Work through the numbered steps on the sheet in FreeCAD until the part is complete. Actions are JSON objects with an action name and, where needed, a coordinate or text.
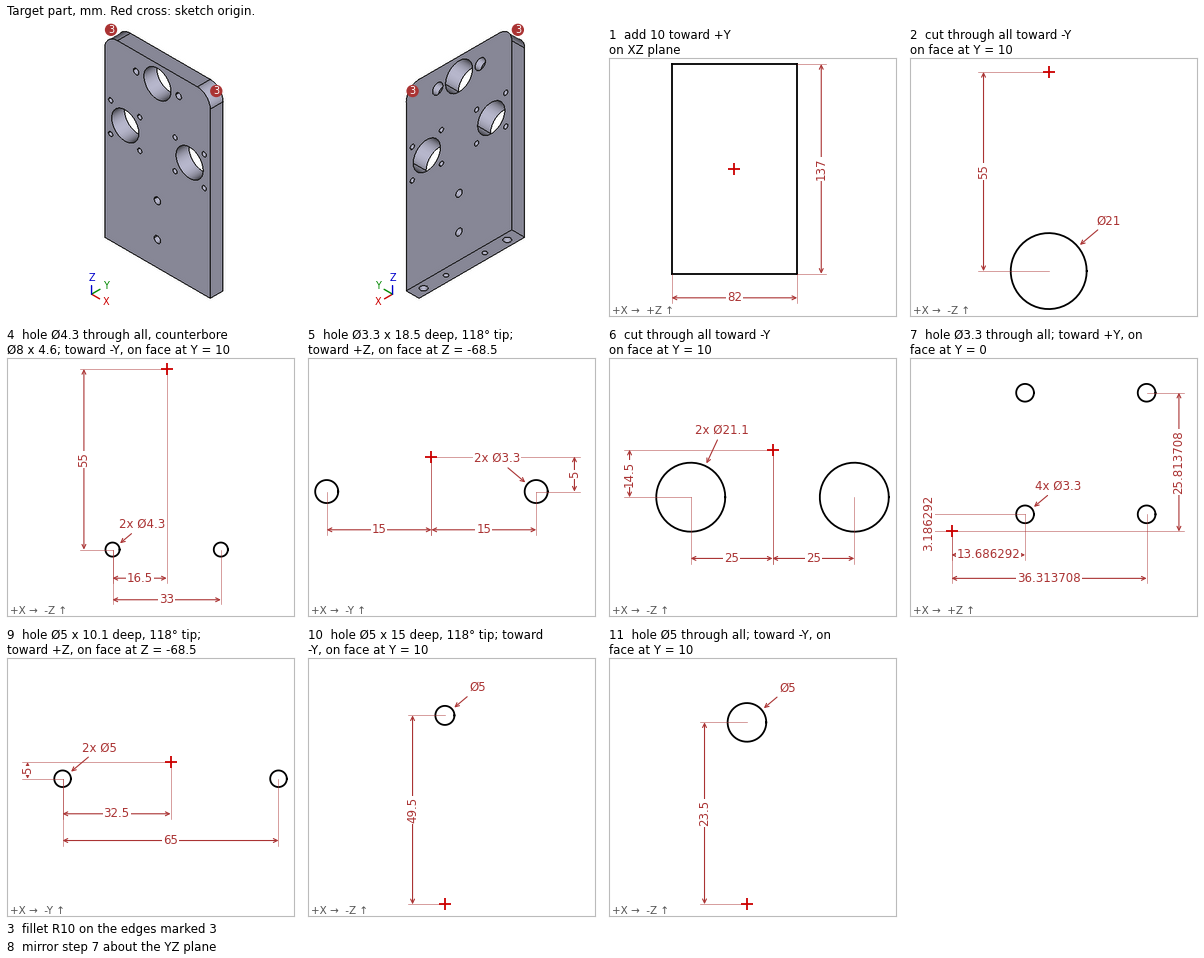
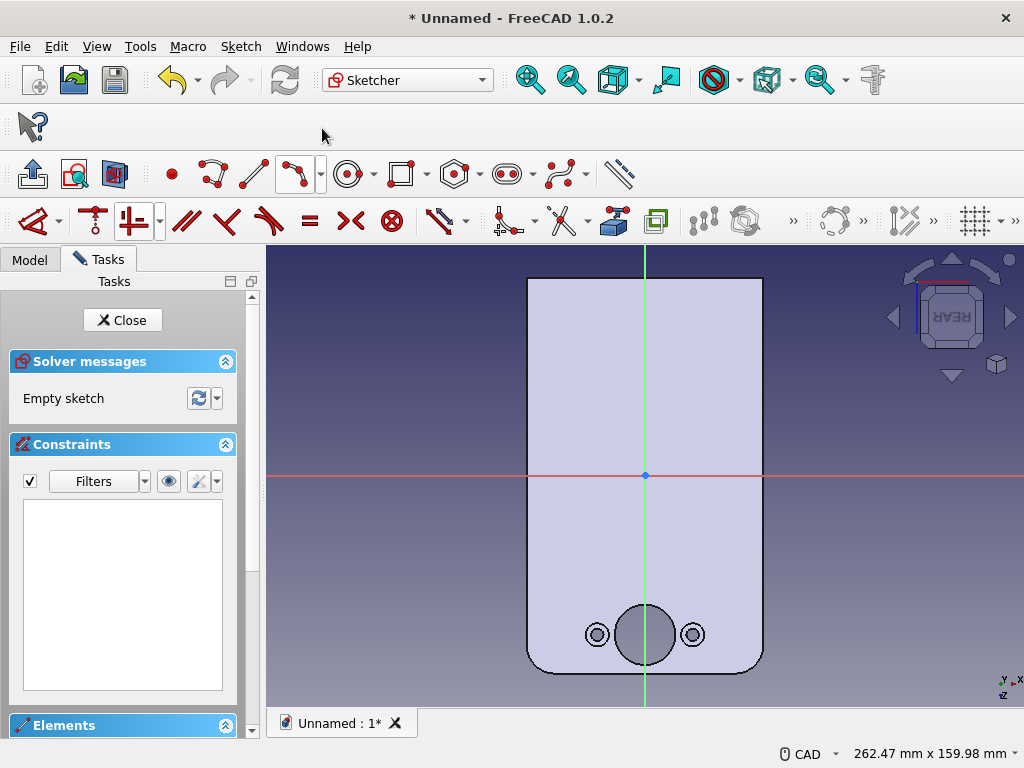
{"action": "scroll", "coordinate": [728, 556], "scroll_direction": "up", "scroll_amount": 3}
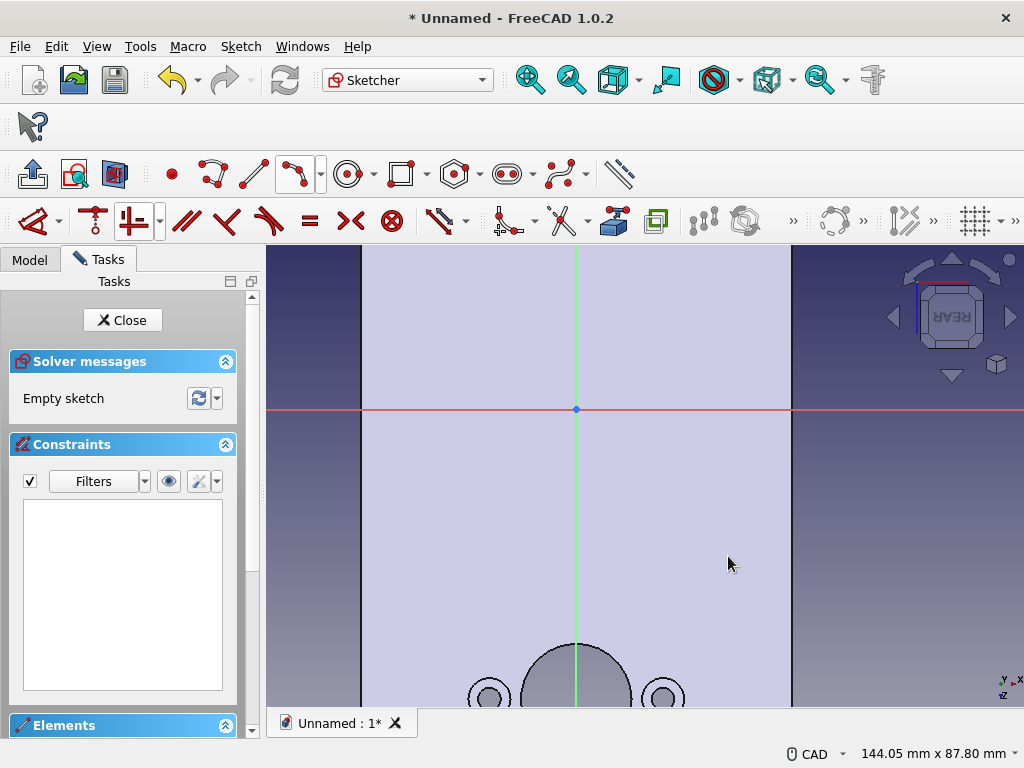
{"action": "key", "text": "g c"}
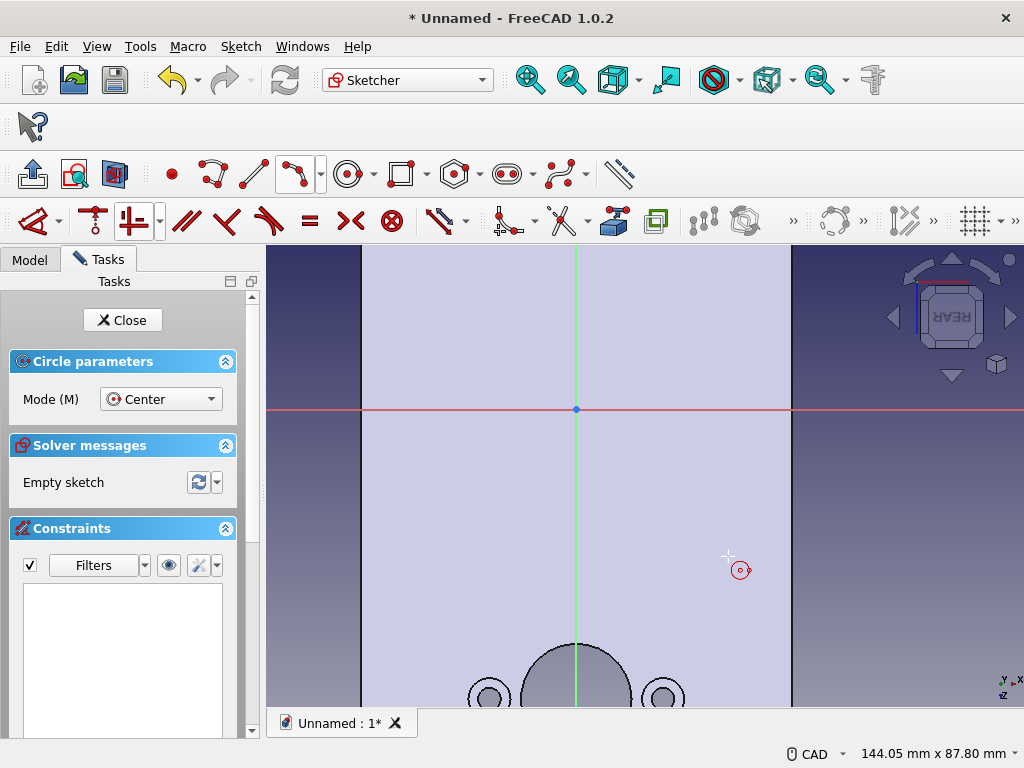
{"action": "left_click", "coordinate": [445, 486]}
{"action": "mouse_move", "coordinate": [484, 447]}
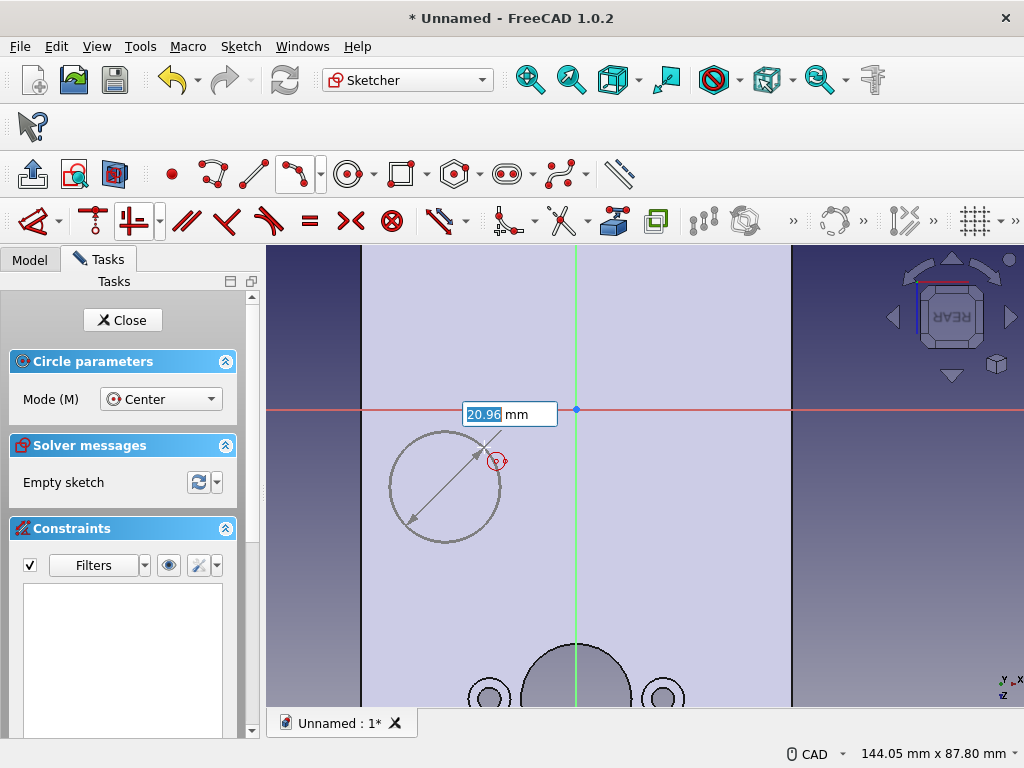
{"action": "type", "text": "21.1"}
{"action": "key", "text": "Return"}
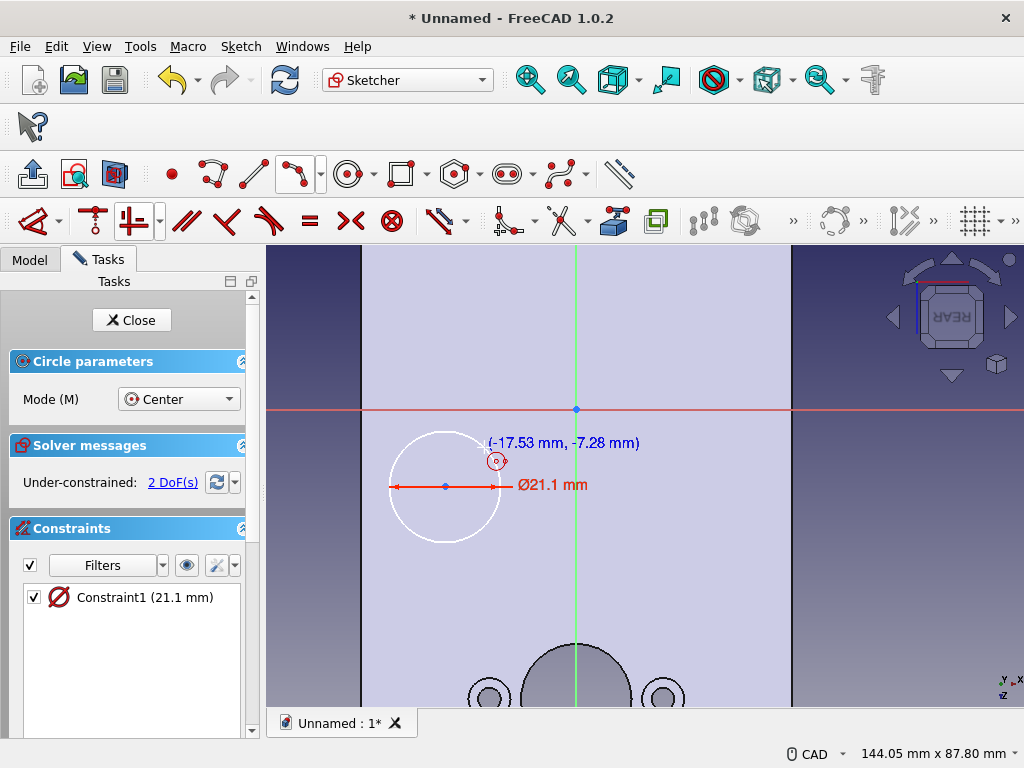
{"action": "left_click", "coordinate": [708, 486]}
{"action": "mouse_move", "coordinate": [747, 447]}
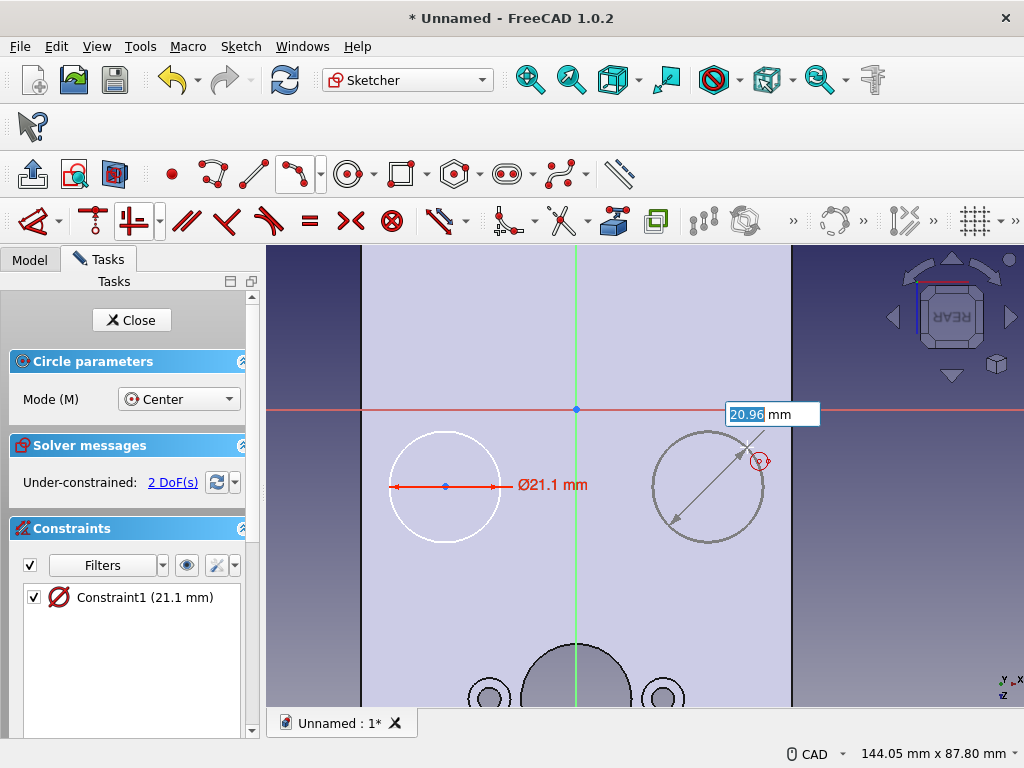
{"action": "type", "text": "21.1"}
{"action": "key", "text": "Return"}
{"action": "key", "text": "Escape"}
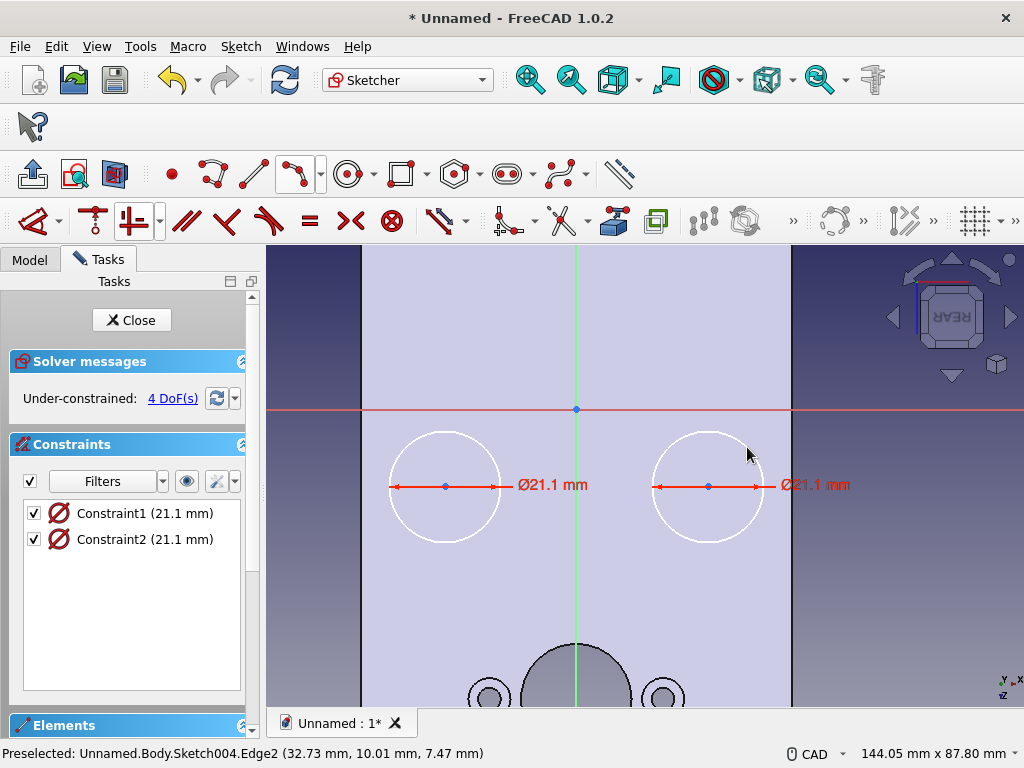
{"action": "left_click", "coordinate": [445, 487]}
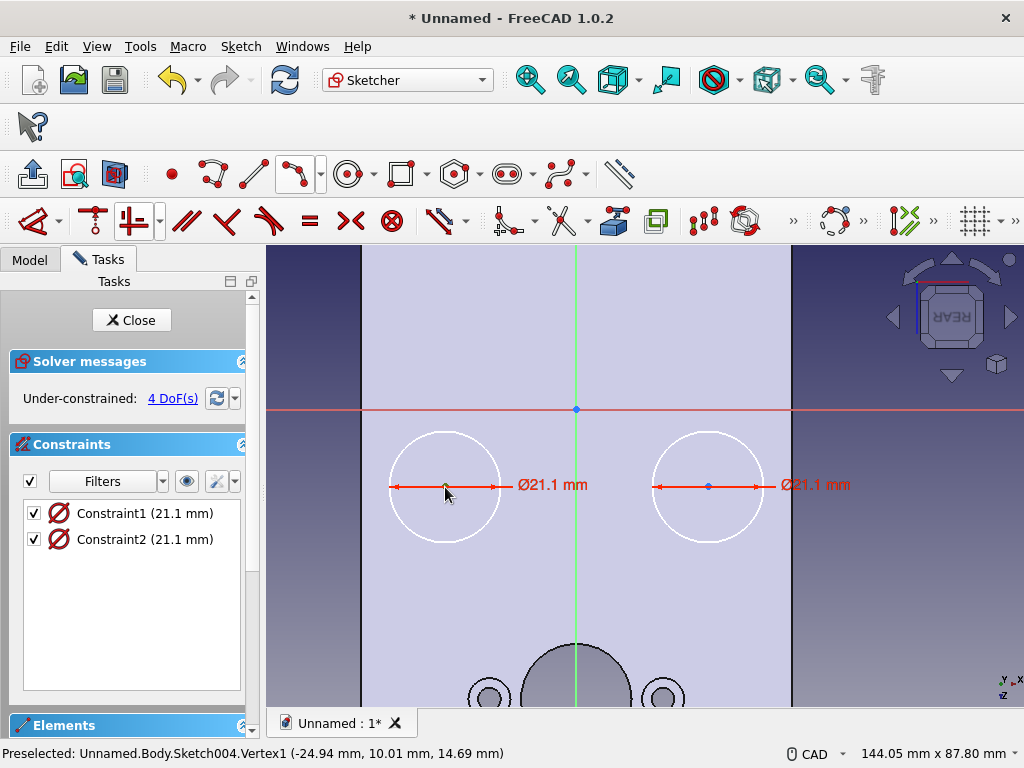
{"action": "left_click", "coordinate": [708, 487]}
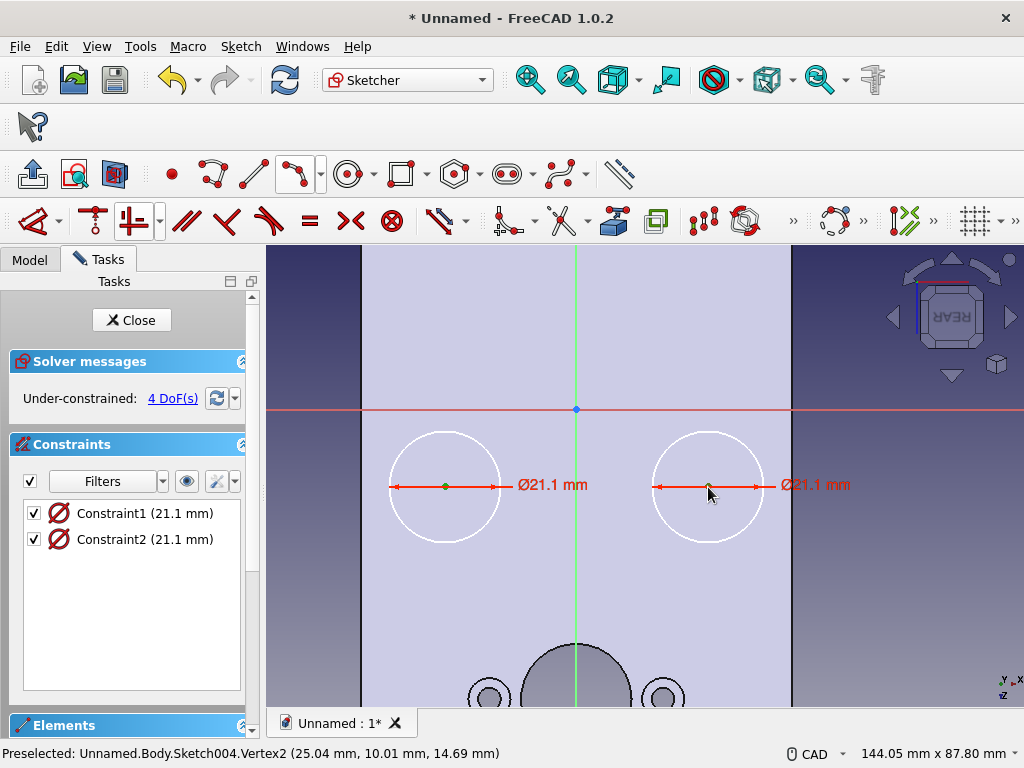
{"action": "key", "text": "h"}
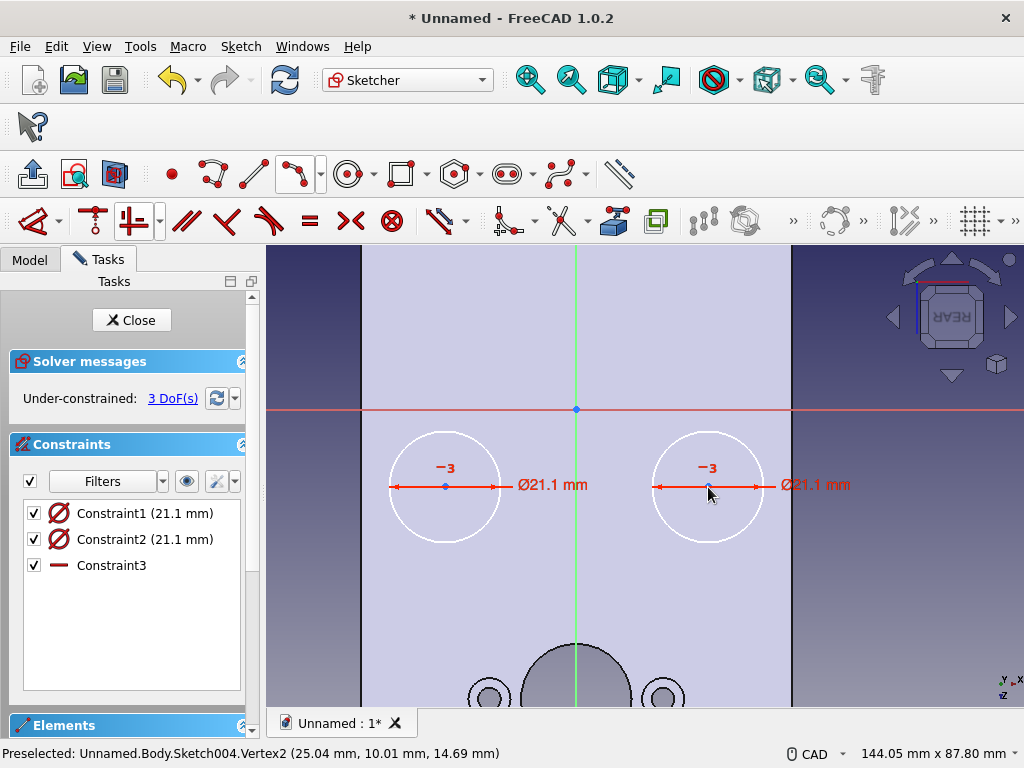
{"action": "key", "text": "d"}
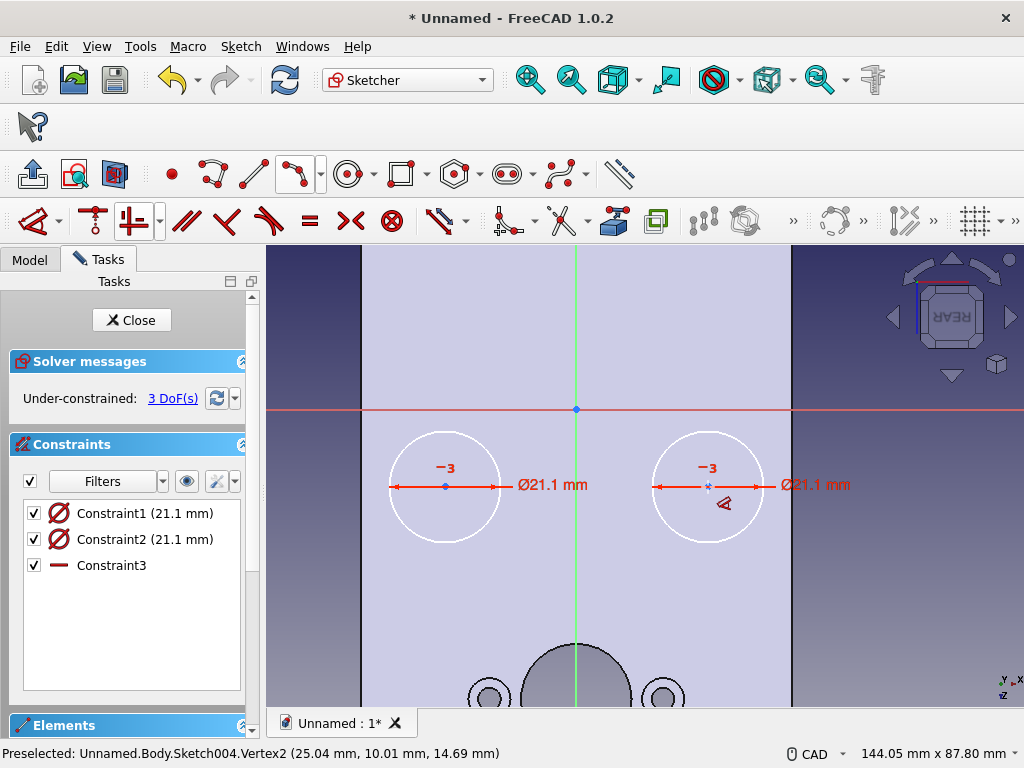
{"action": "left_click", "coordinate": [445, 487]}
{"action": "left_click", "coordinate": [511, 376]}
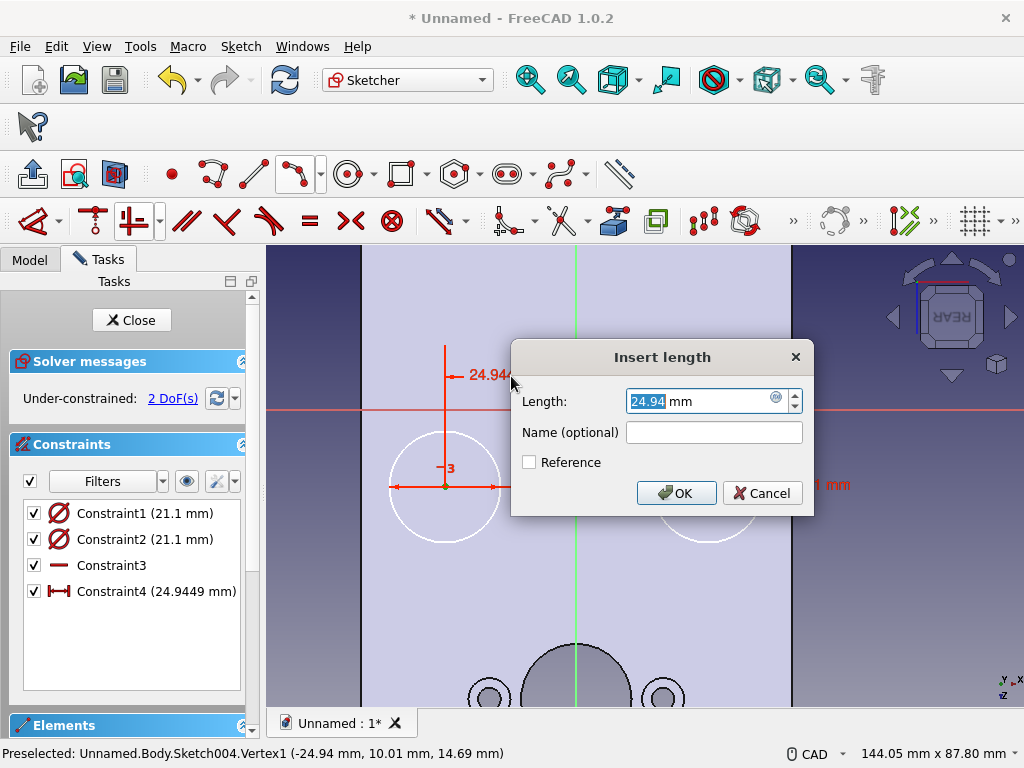
{"action": "type", "text": "25"}
{"action": "key", "text": "Return"}